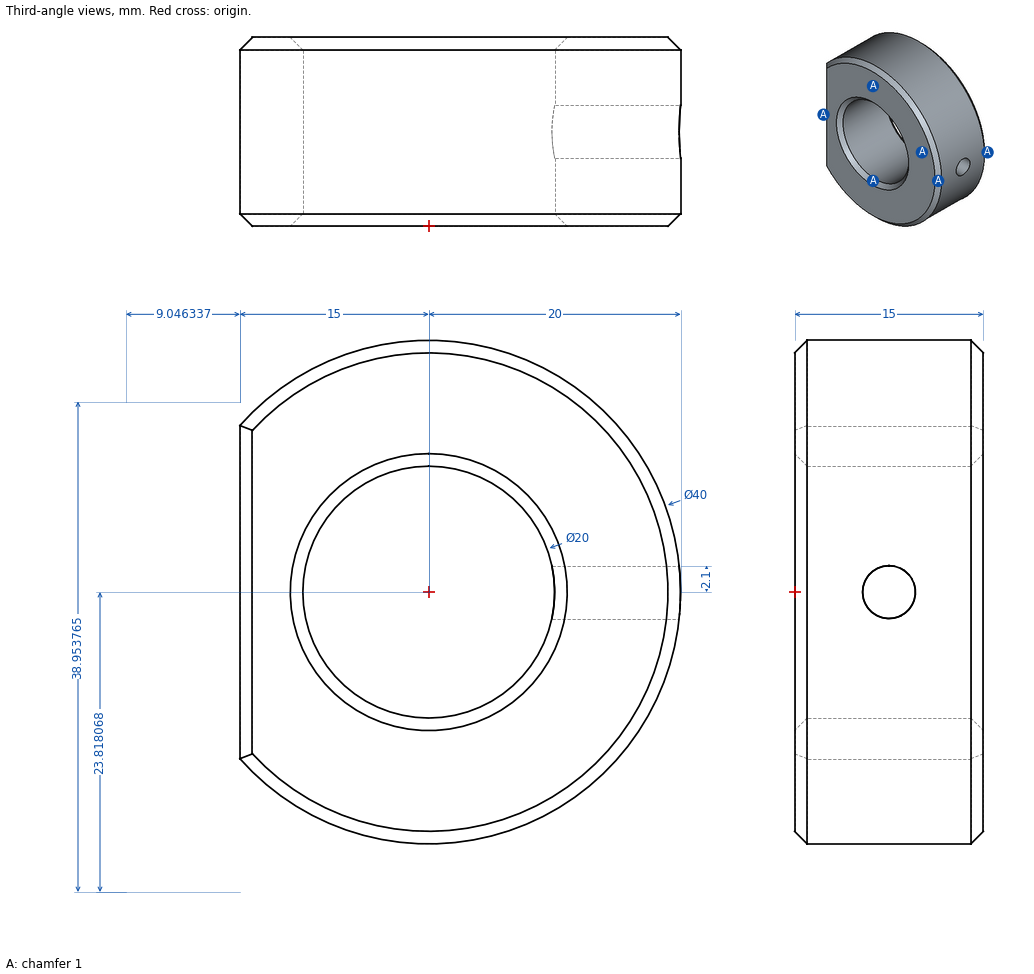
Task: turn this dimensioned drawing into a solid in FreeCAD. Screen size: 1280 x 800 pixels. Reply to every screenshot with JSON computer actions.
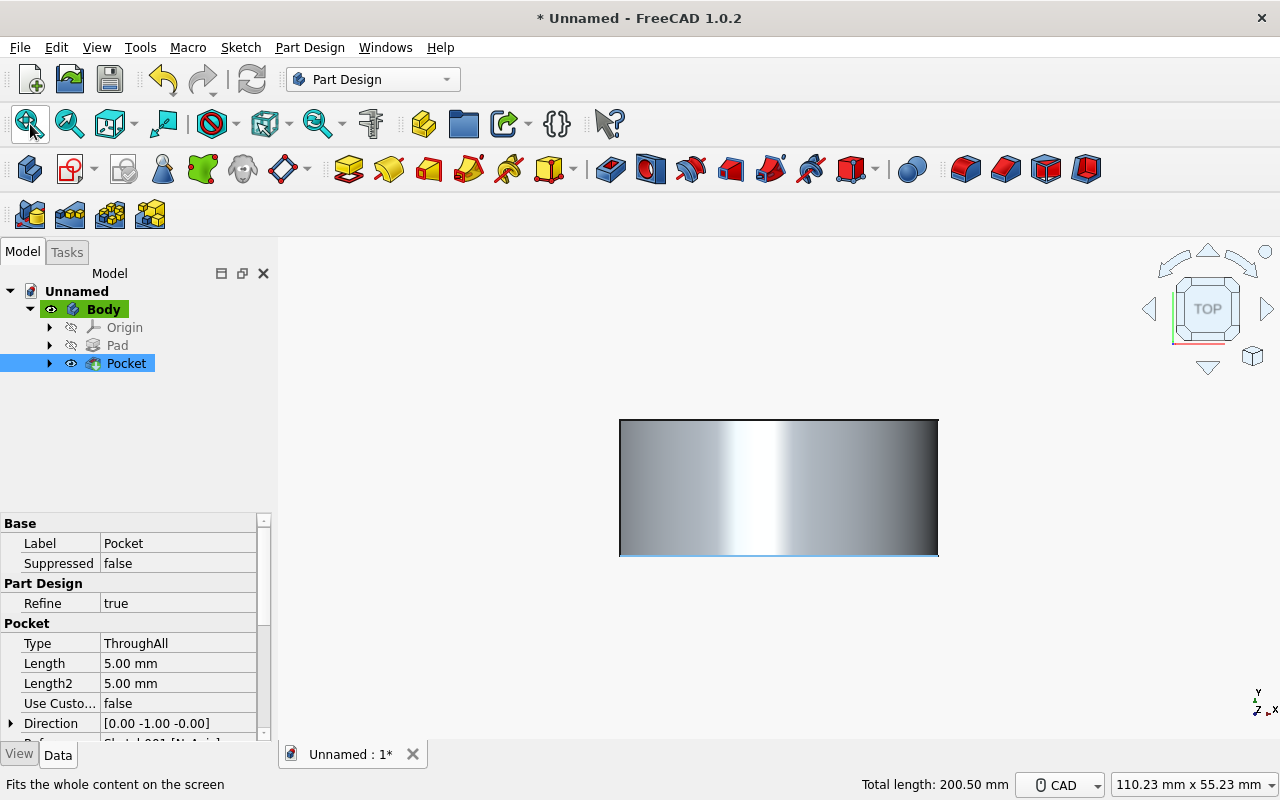
{"action": "left_click", "coordinate": [821, 419], "text": "ctrl"}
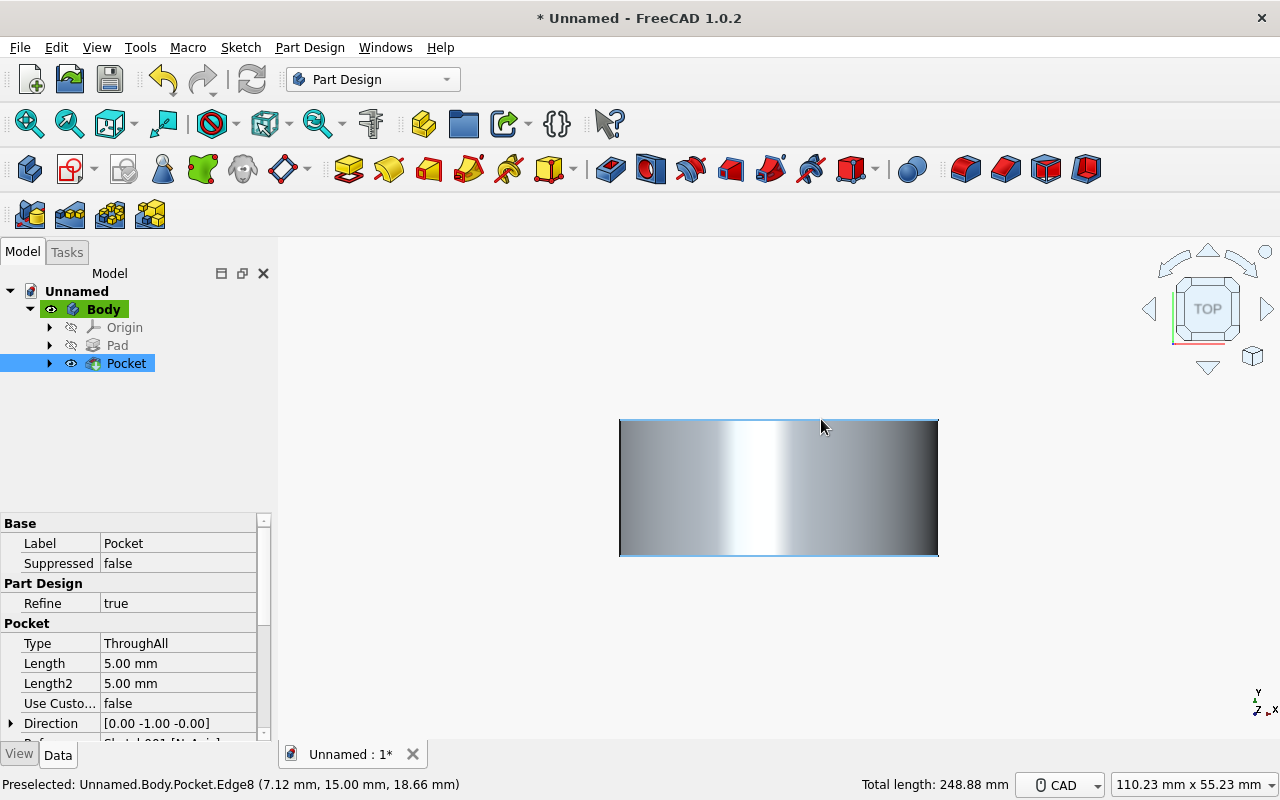
{"action": "key", "text": "1"}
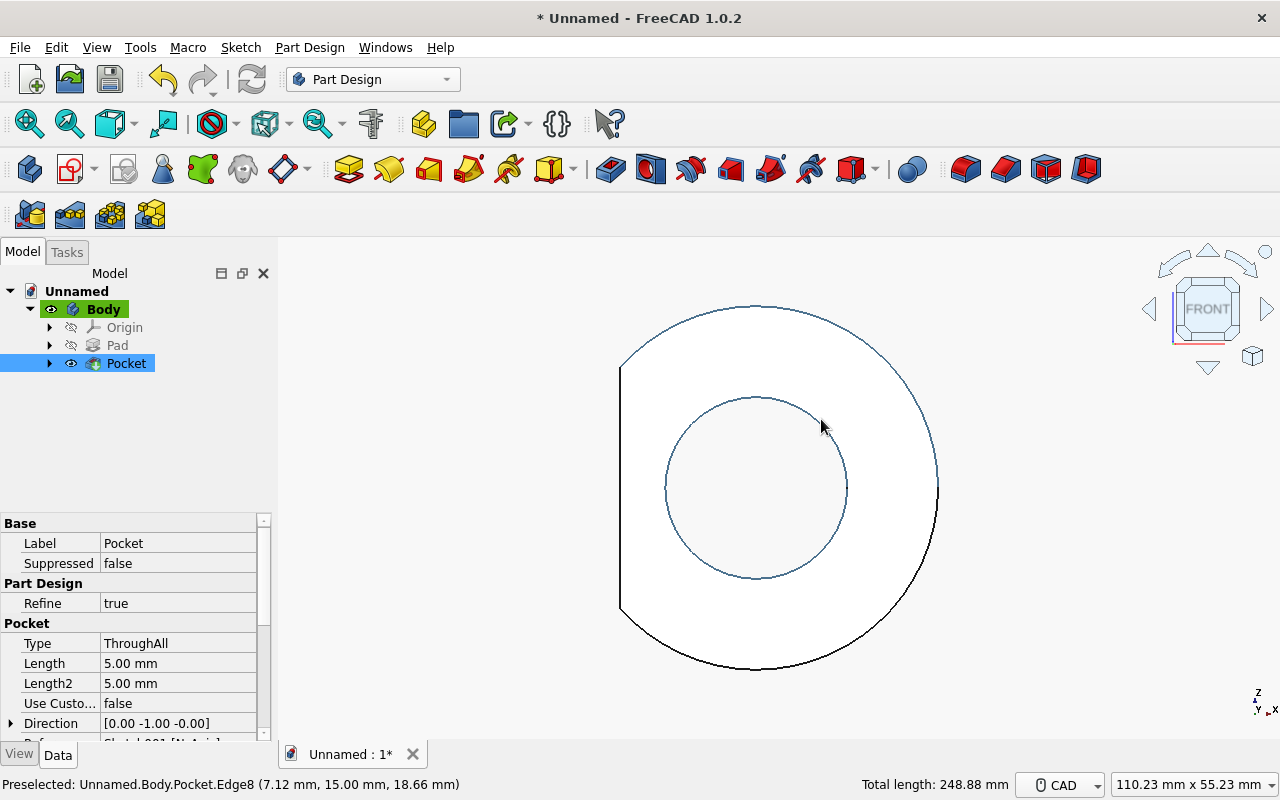
{"action": "key", "text": "3"}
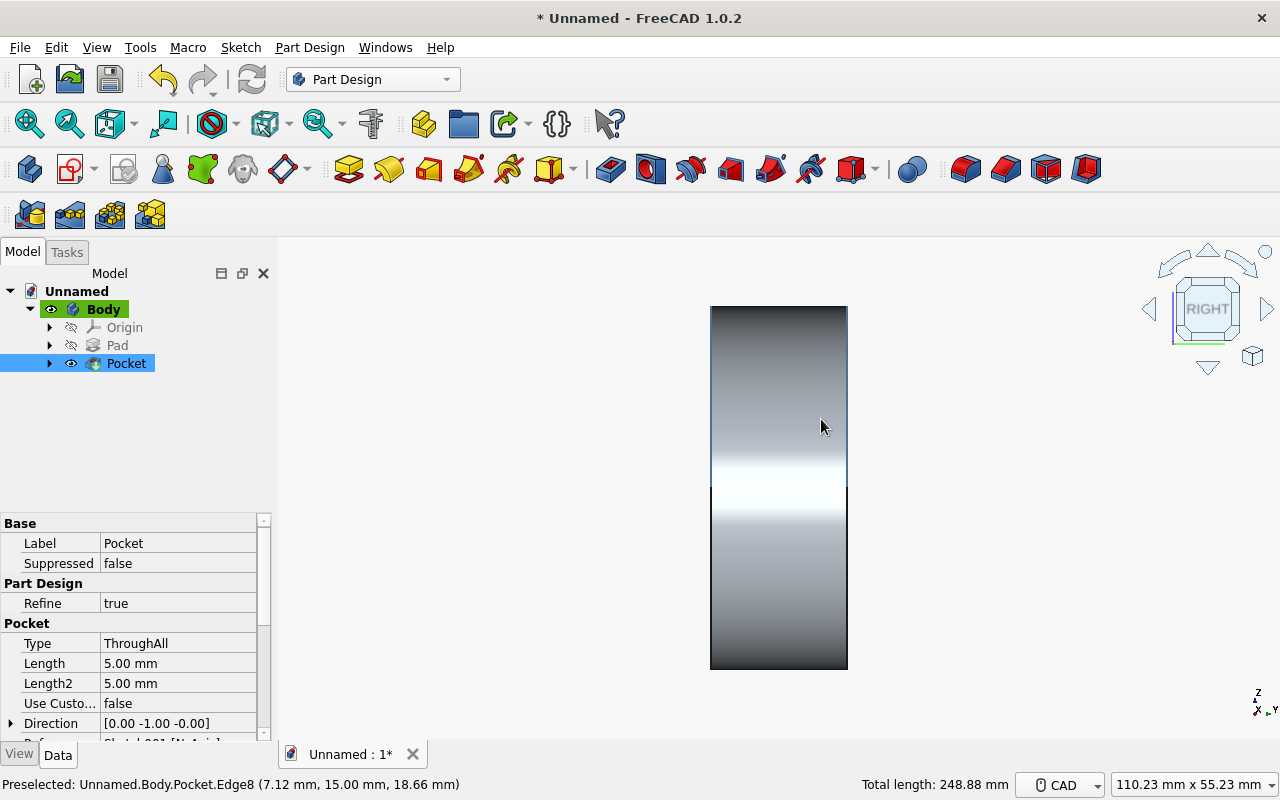
{"action": "key", "text": "5"}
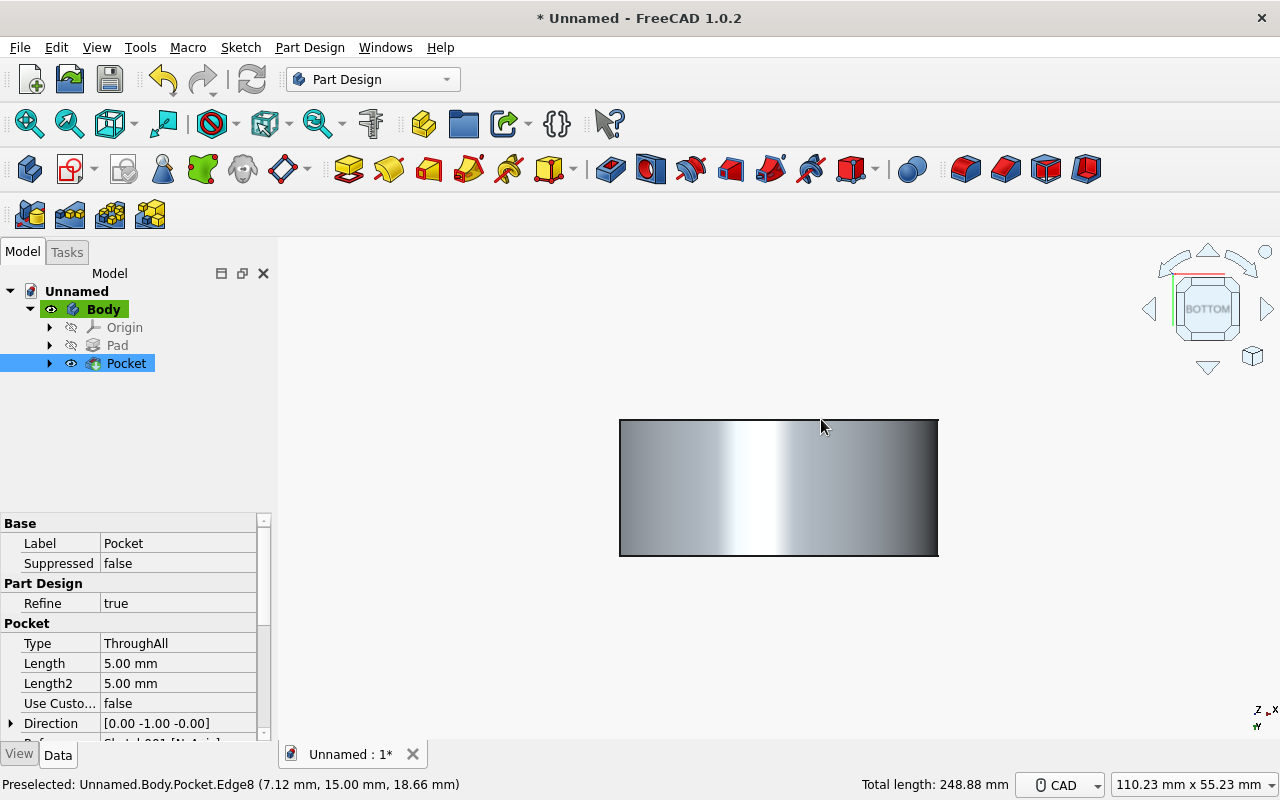
{"action": "key", "text": "v f"}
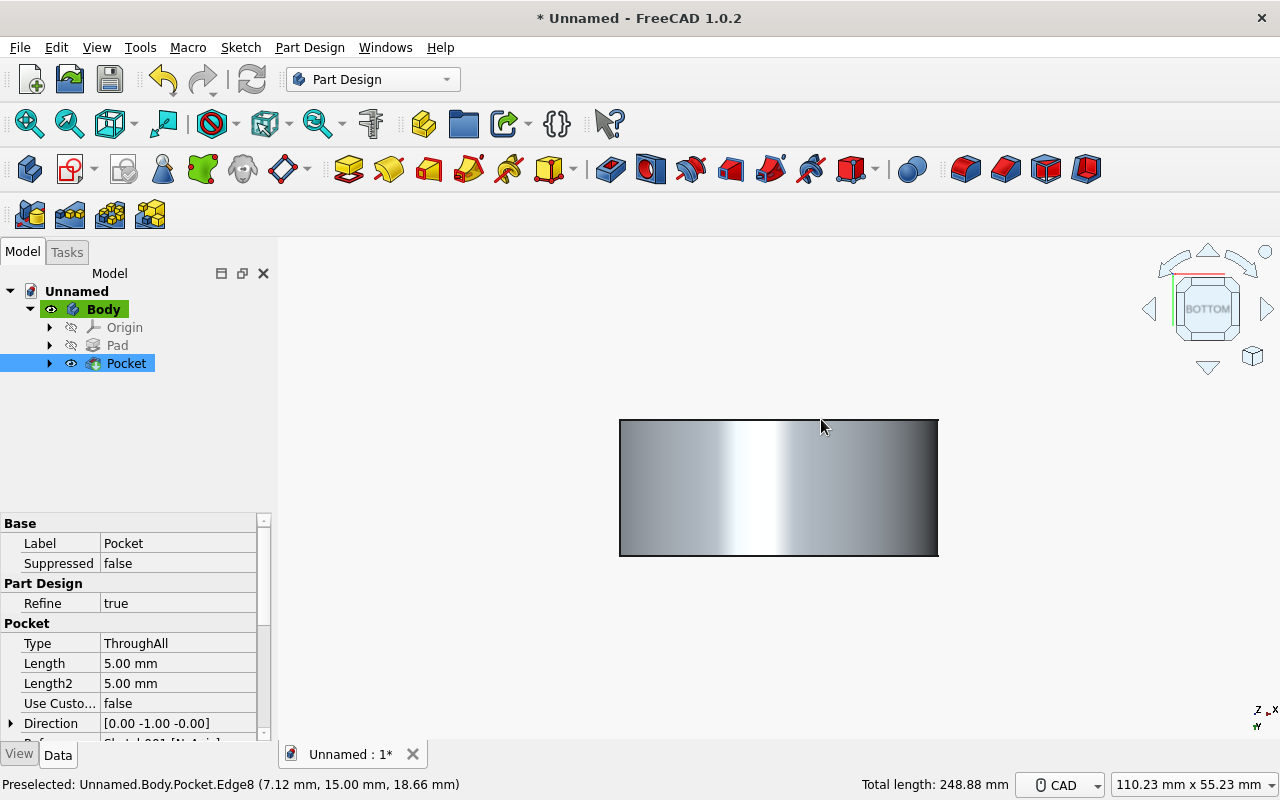
{"action": "key", "text": "4"}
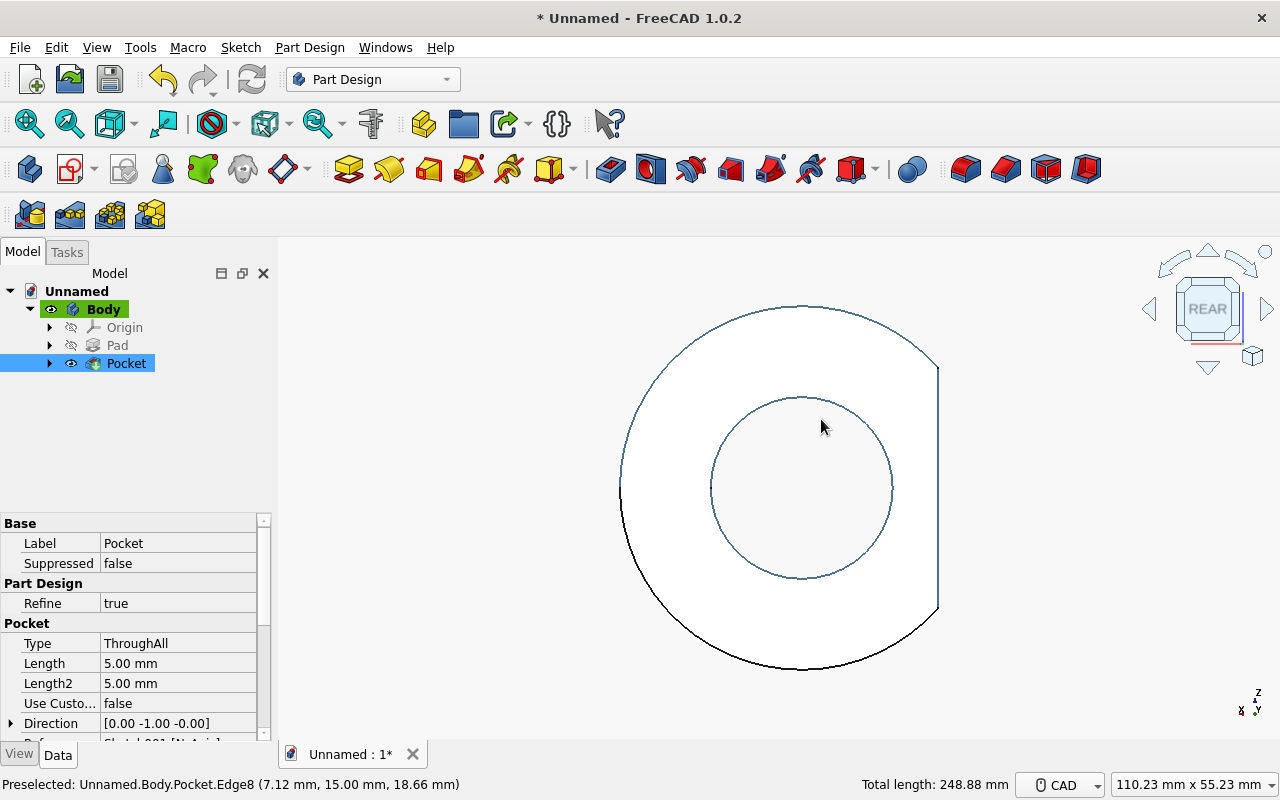
{"action": "key", "text": "6"}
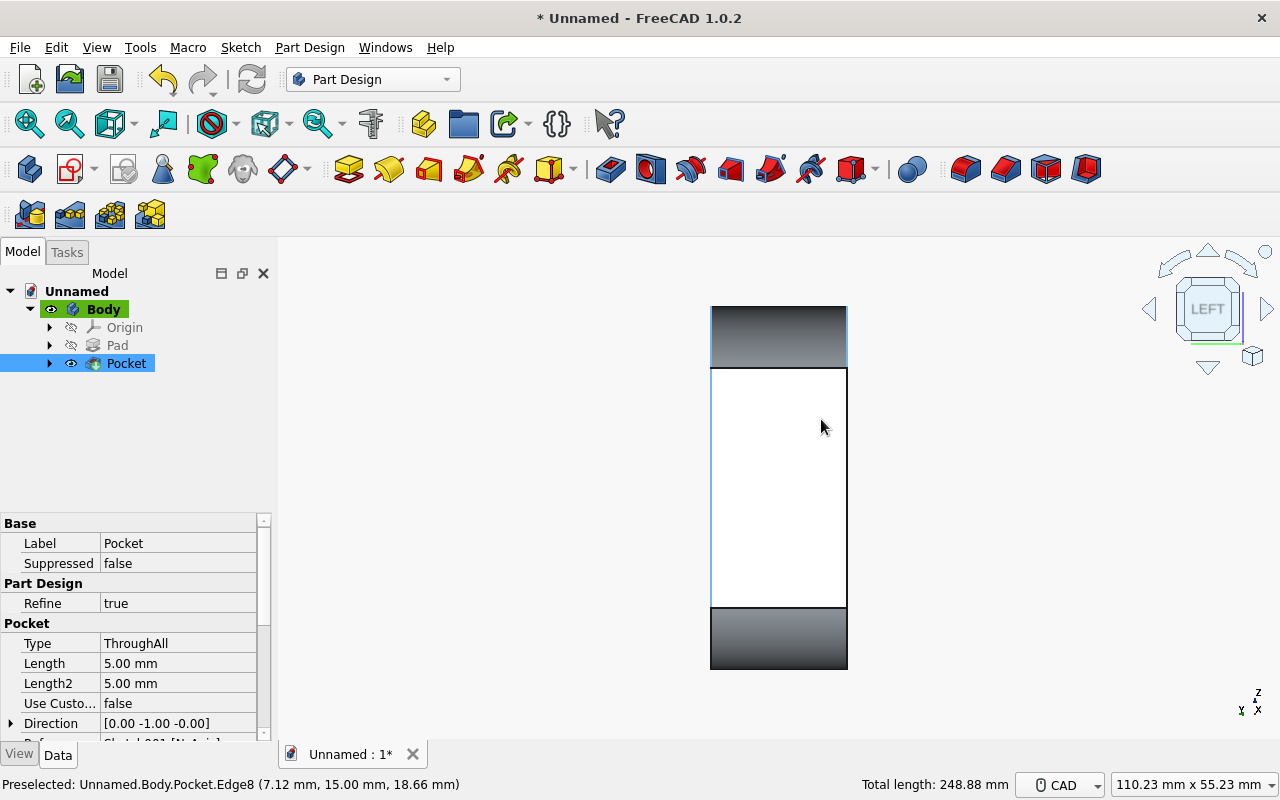
{"action": "left_click", "coordinate": [847, 487], "text": "ctrl"}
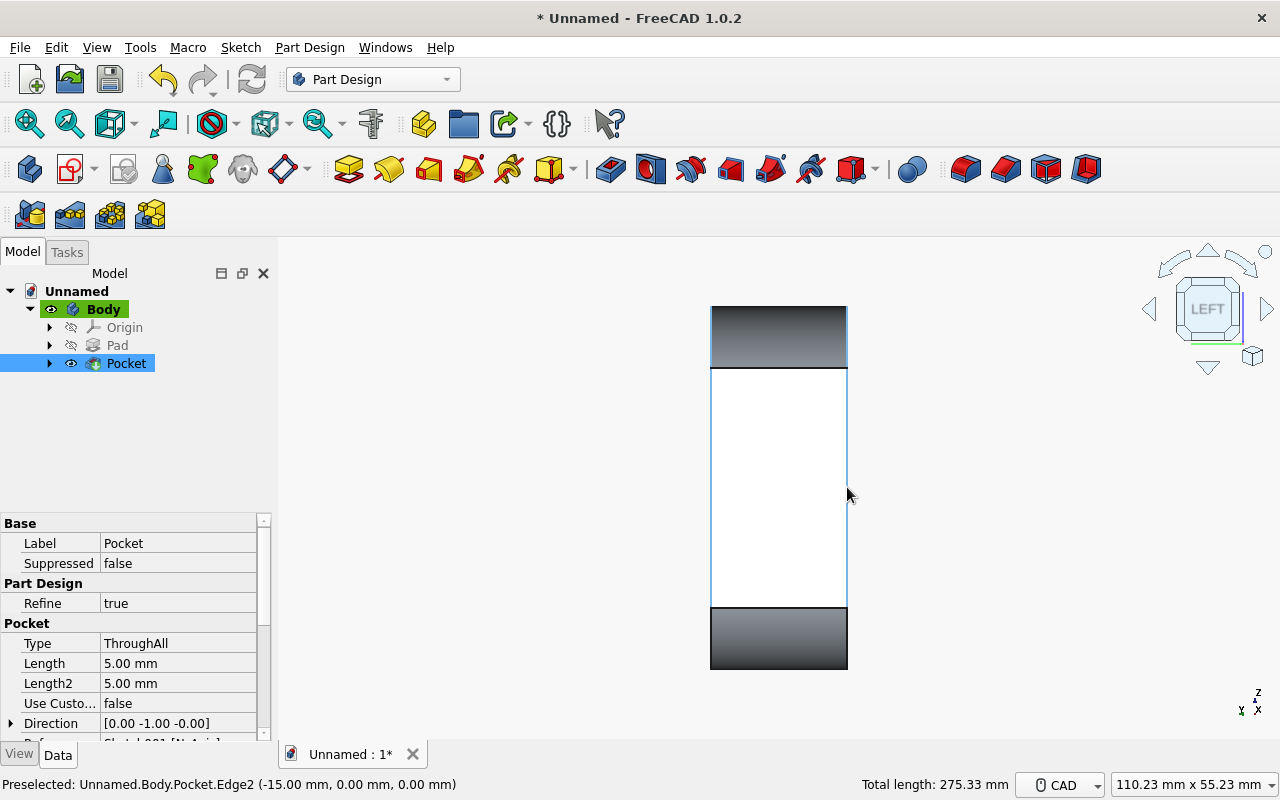
{"action": "left_click", "coordinate": [1006, 170]}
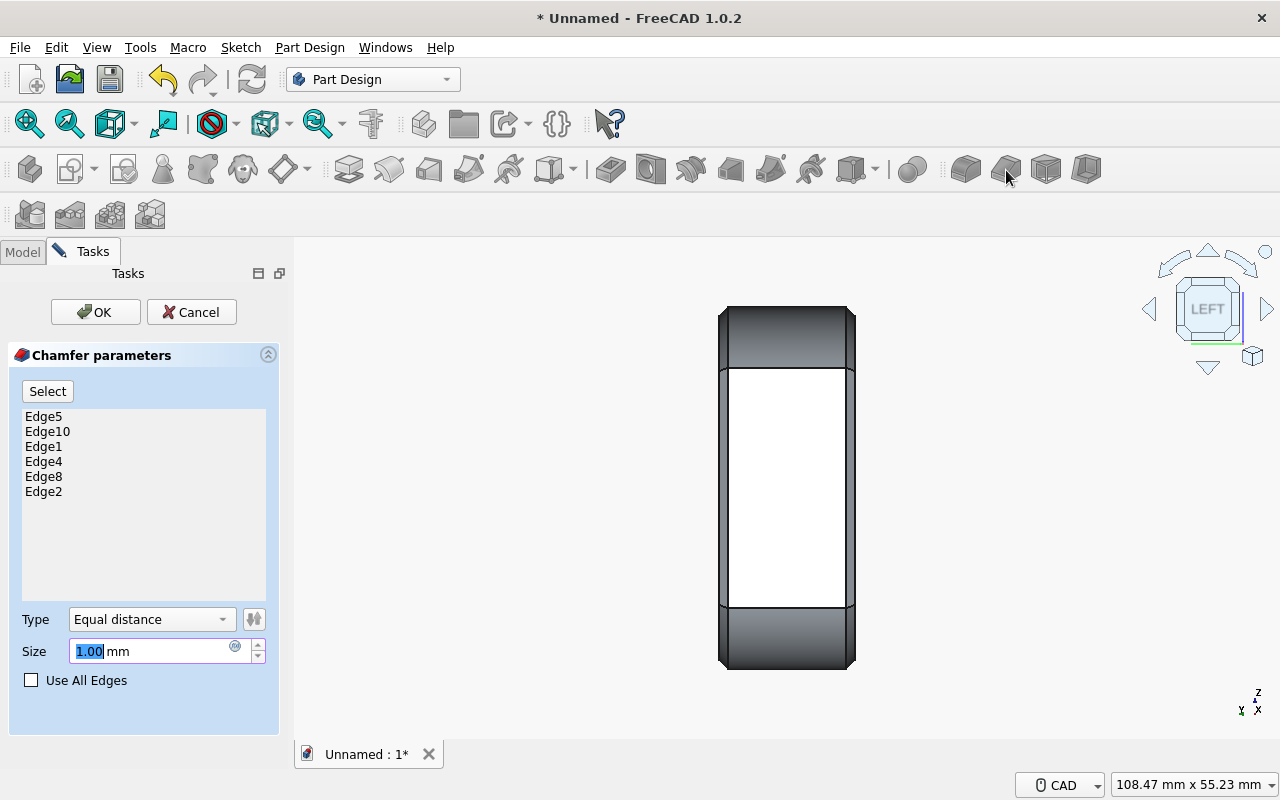
{"action": "type", "text": "1"}
{"action": "key", "text": "Tab"}